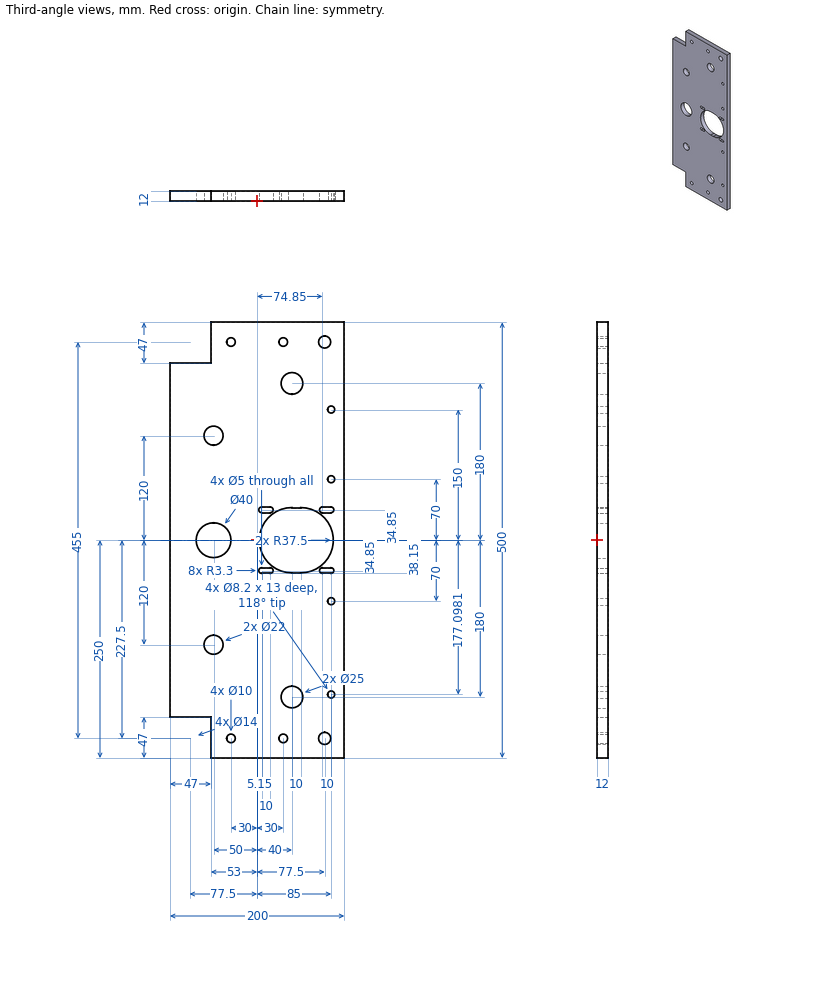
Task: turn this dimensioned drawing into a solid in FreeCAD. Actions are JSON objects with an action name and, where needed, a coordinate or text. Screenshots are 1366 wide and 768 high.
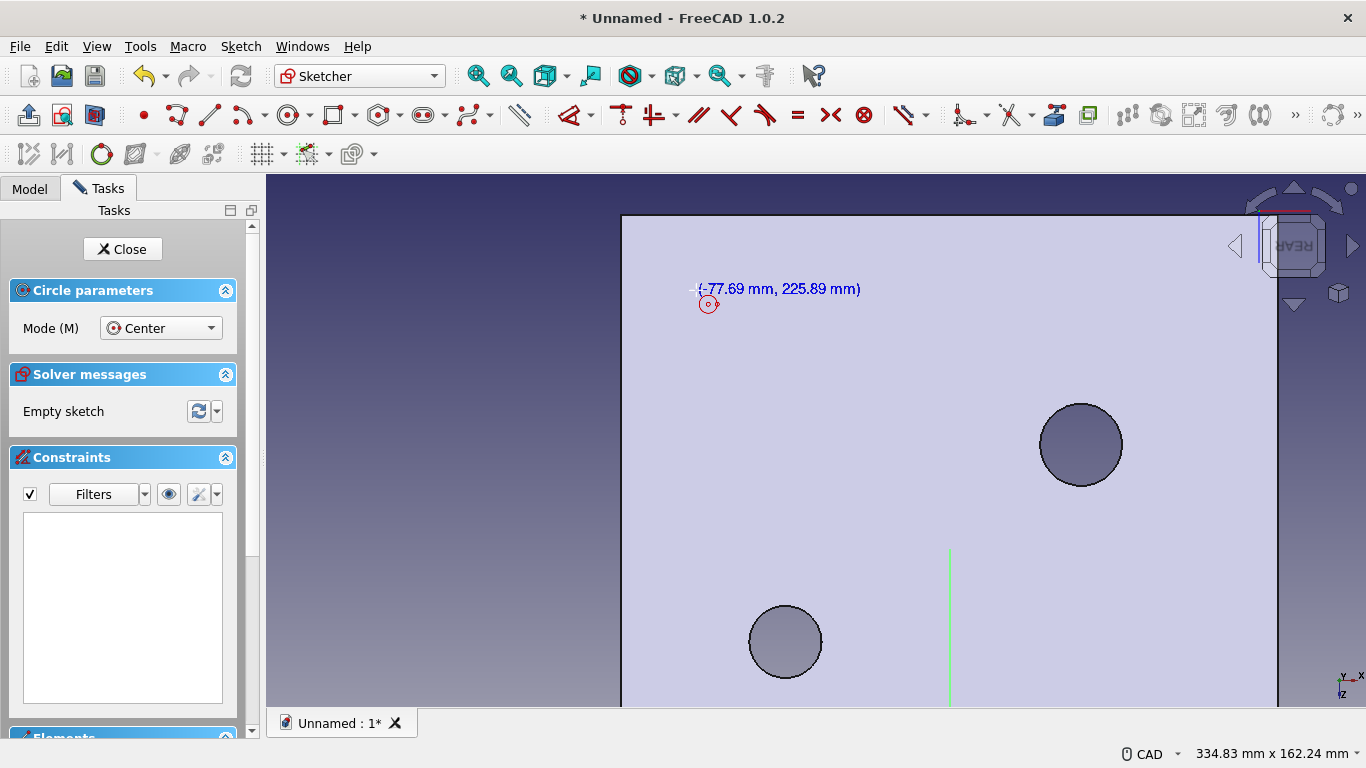
{"action": "scroll", "coordinate": [696, 290], "scroll_direction": "down", "scroll_amount": 8}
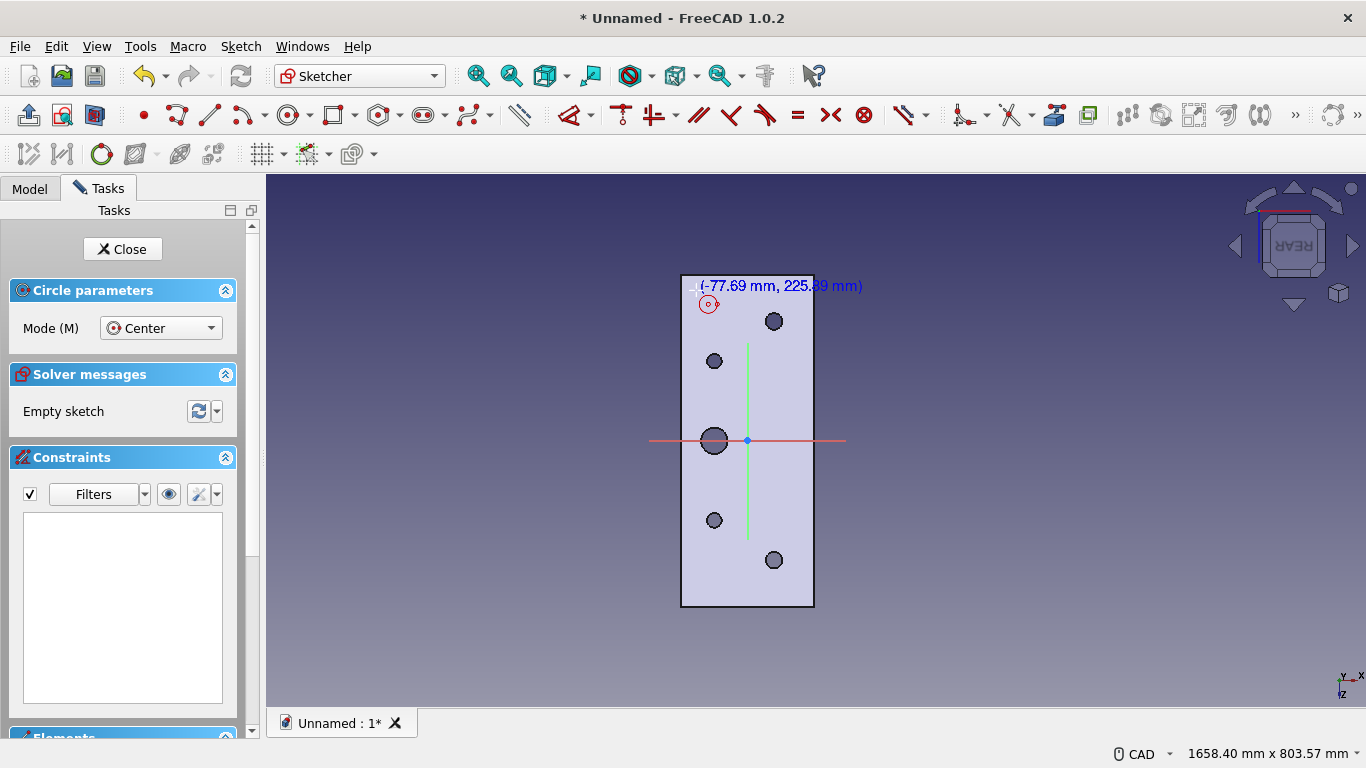
{"action": "left_click", "coordinate": [696, 290]}
{"action": "mouse_move", "coordinate": [699, 287]}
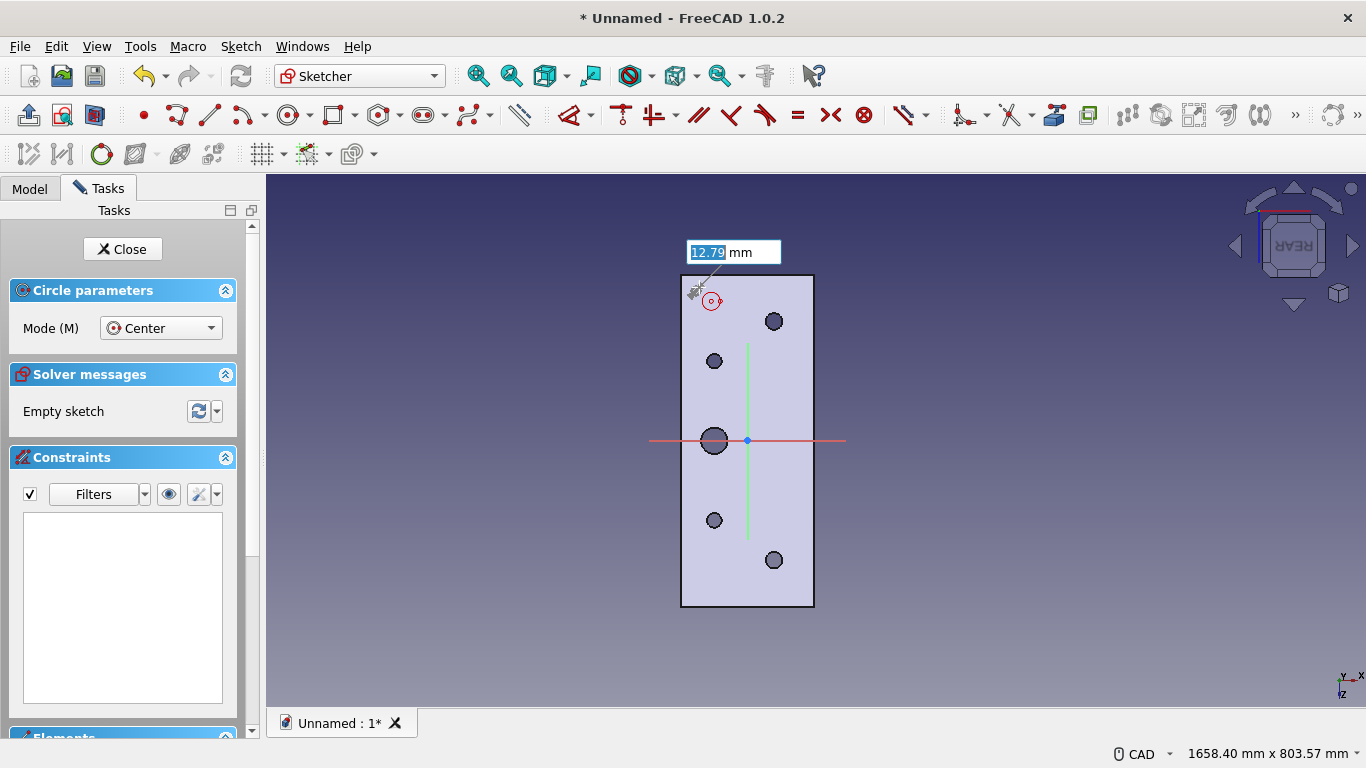
{"action": "type", "text": "14"}
{"action": "key", "text": "Return"}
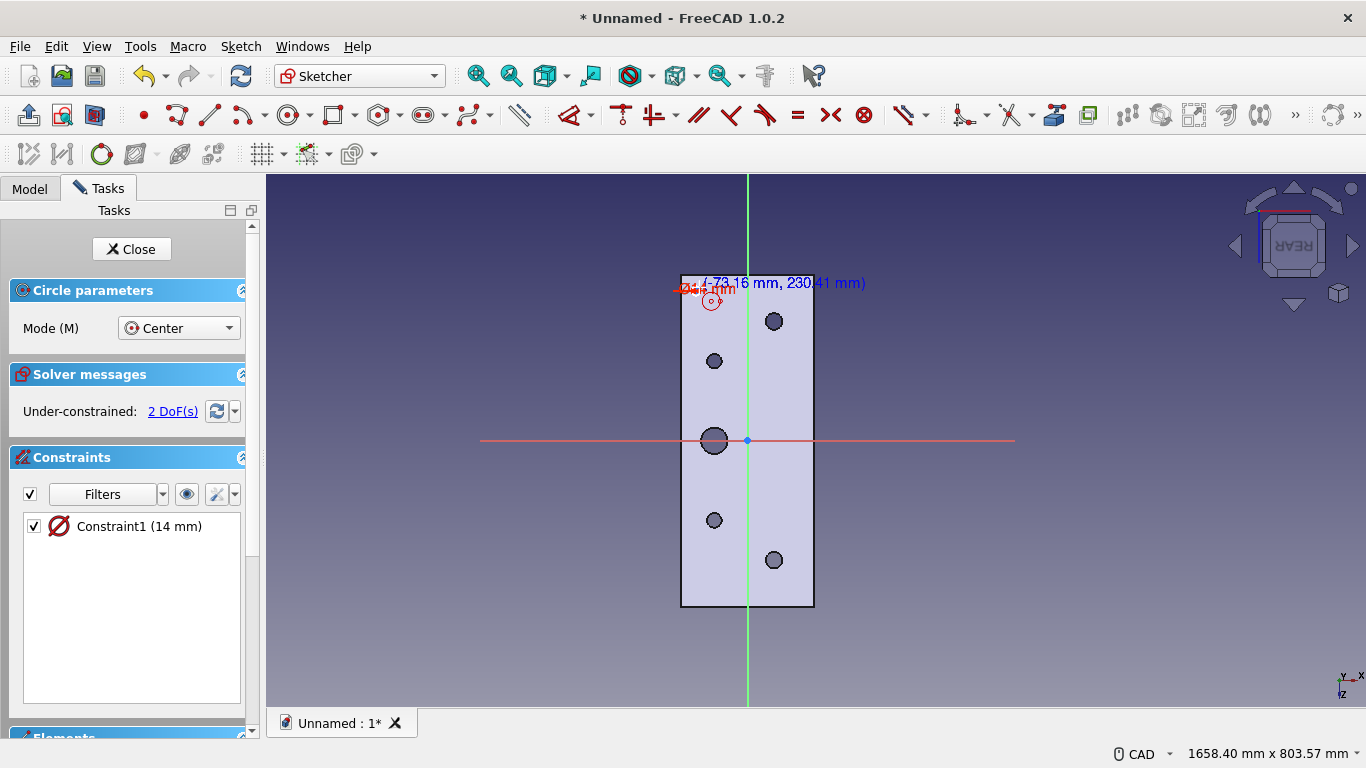
{"action": "scroll", "coordinate": [799, 290], "scroll_direction": "up", "scroll_amount": 8}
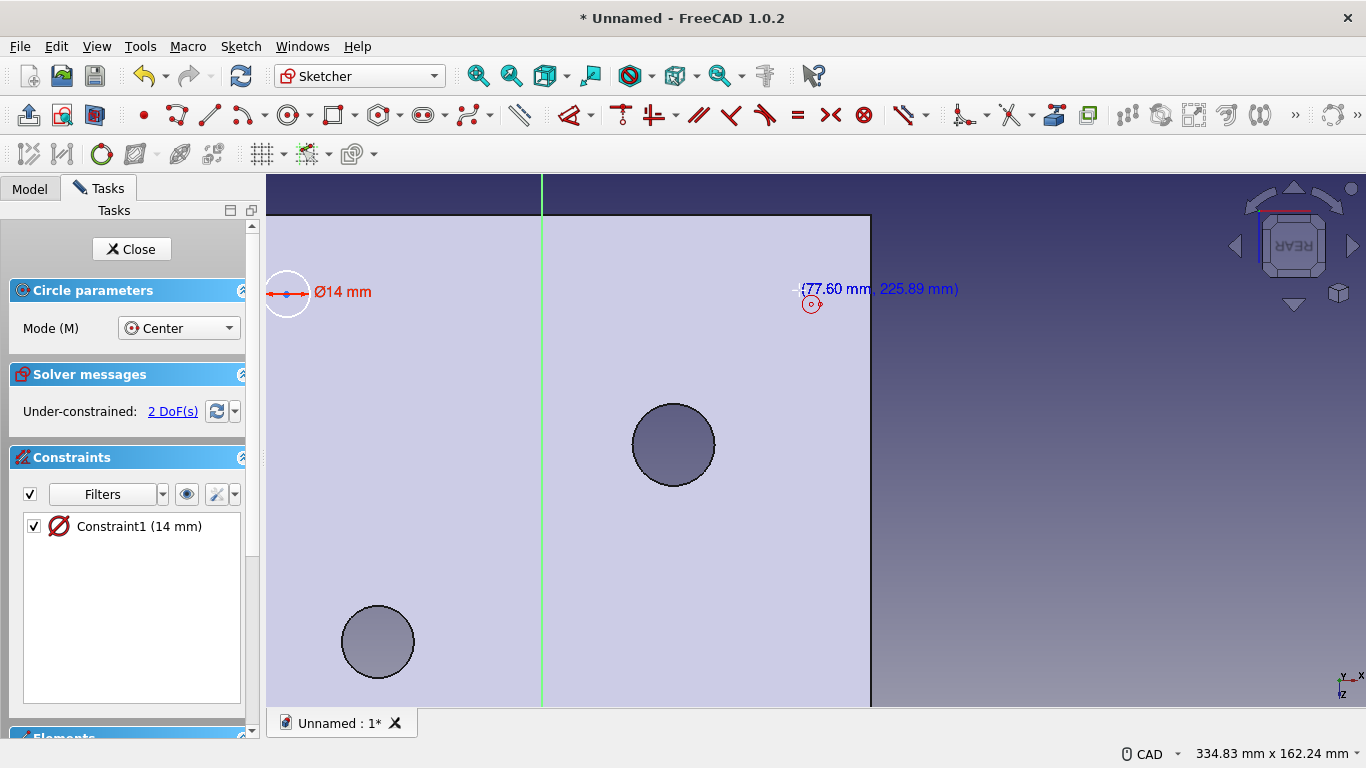
{"action": "scroll", "coordinate": [799, 290], "scroll_direction": "down", "scroll_amount": 8}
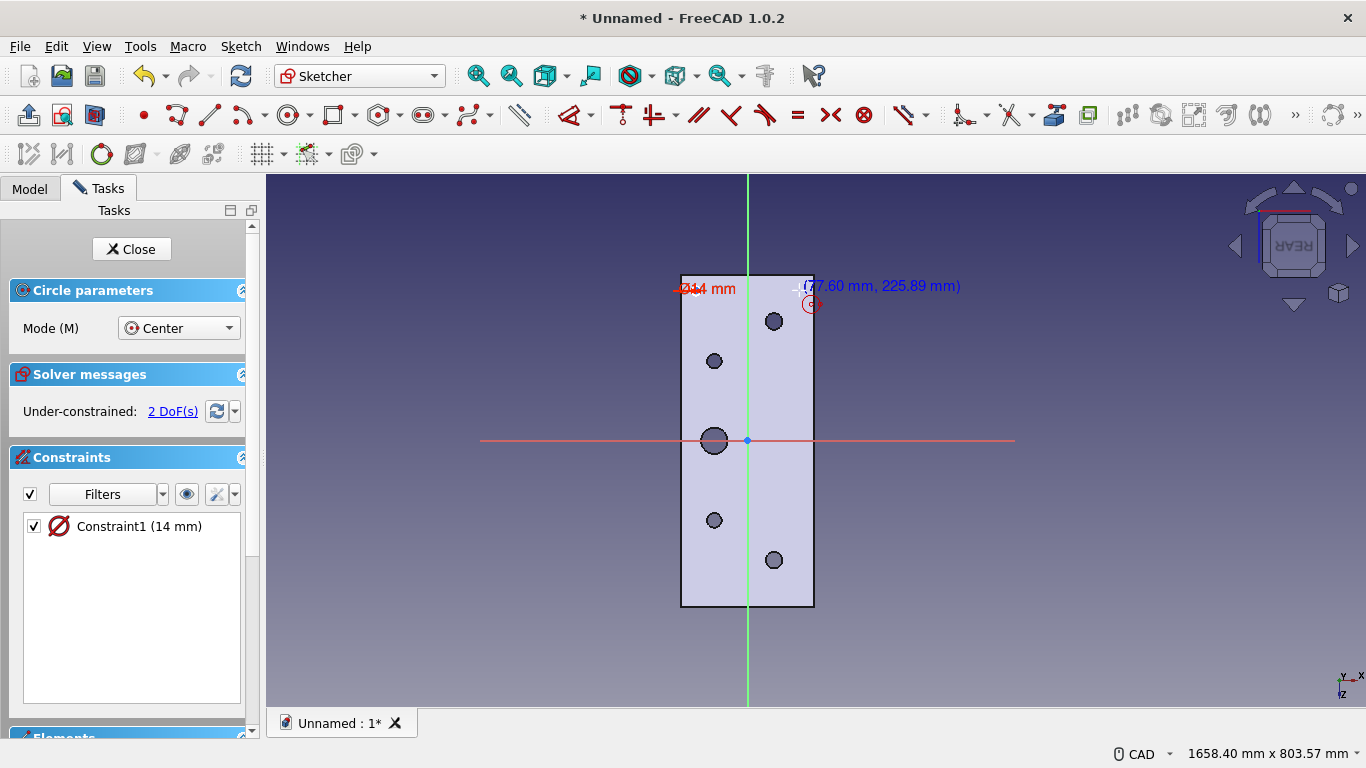
{"action": "left_click", "coordinate": [799, 290]}
{"action": "mouse_move", "coordinate": [802, 287]}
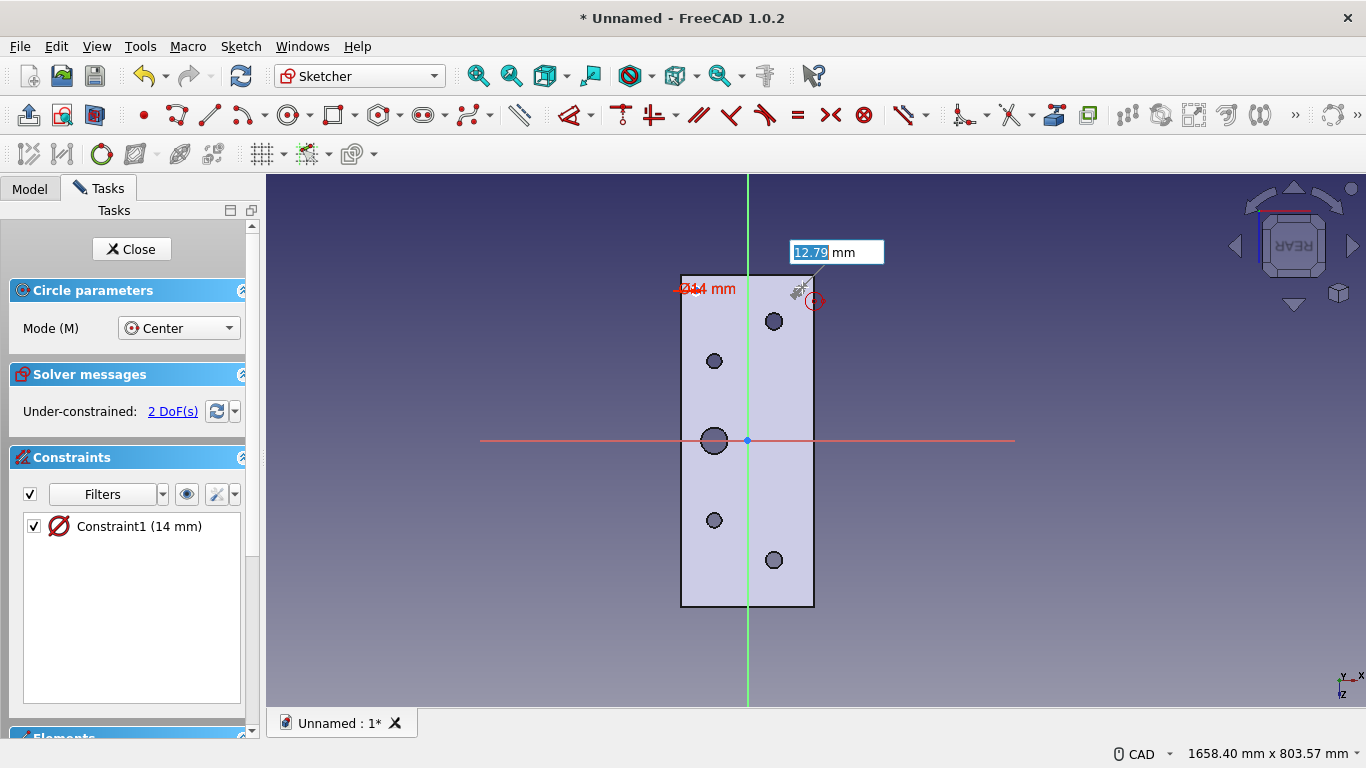
{"action": "type", "text": "14"}
{"action": "key", "text": "Return"}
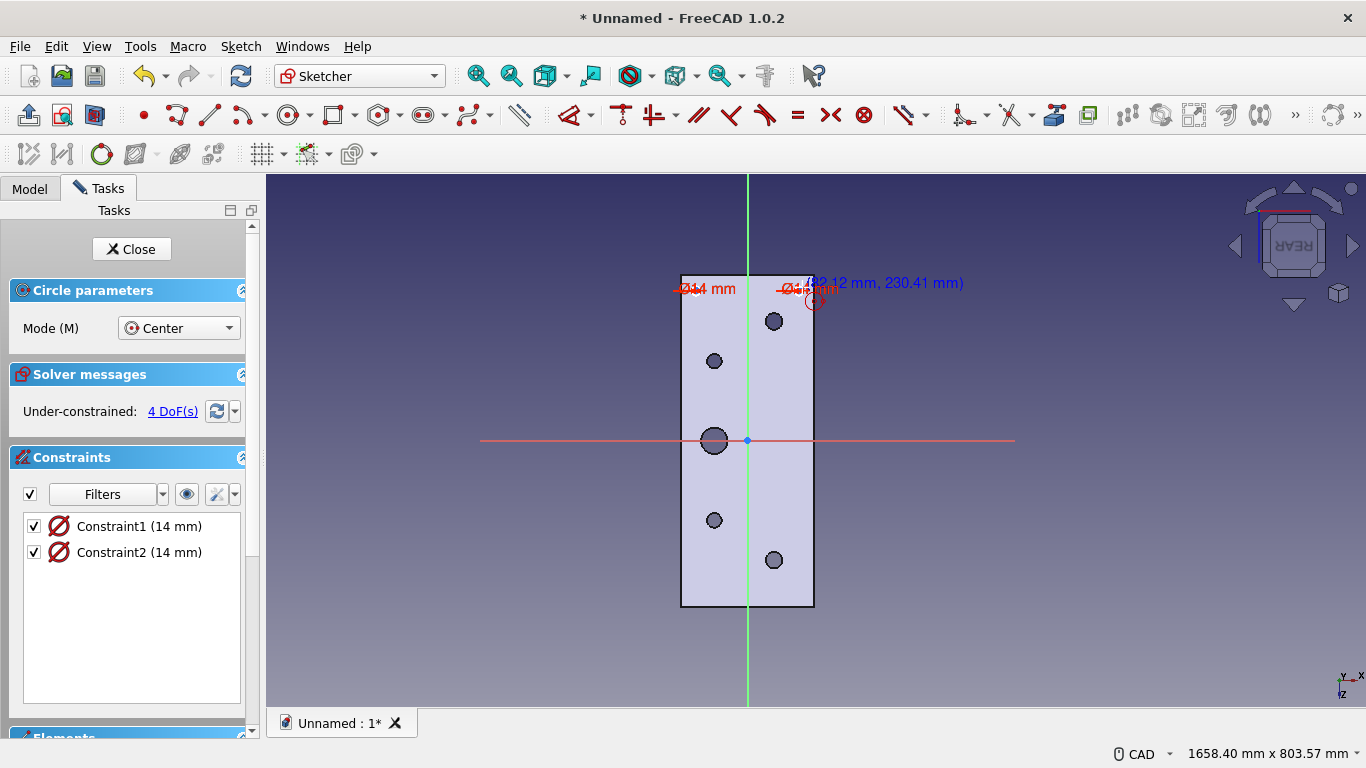
{"action": "scroll", "coordinate": [696, 592], "scroll_direction": "up", "scroll_amount": 8}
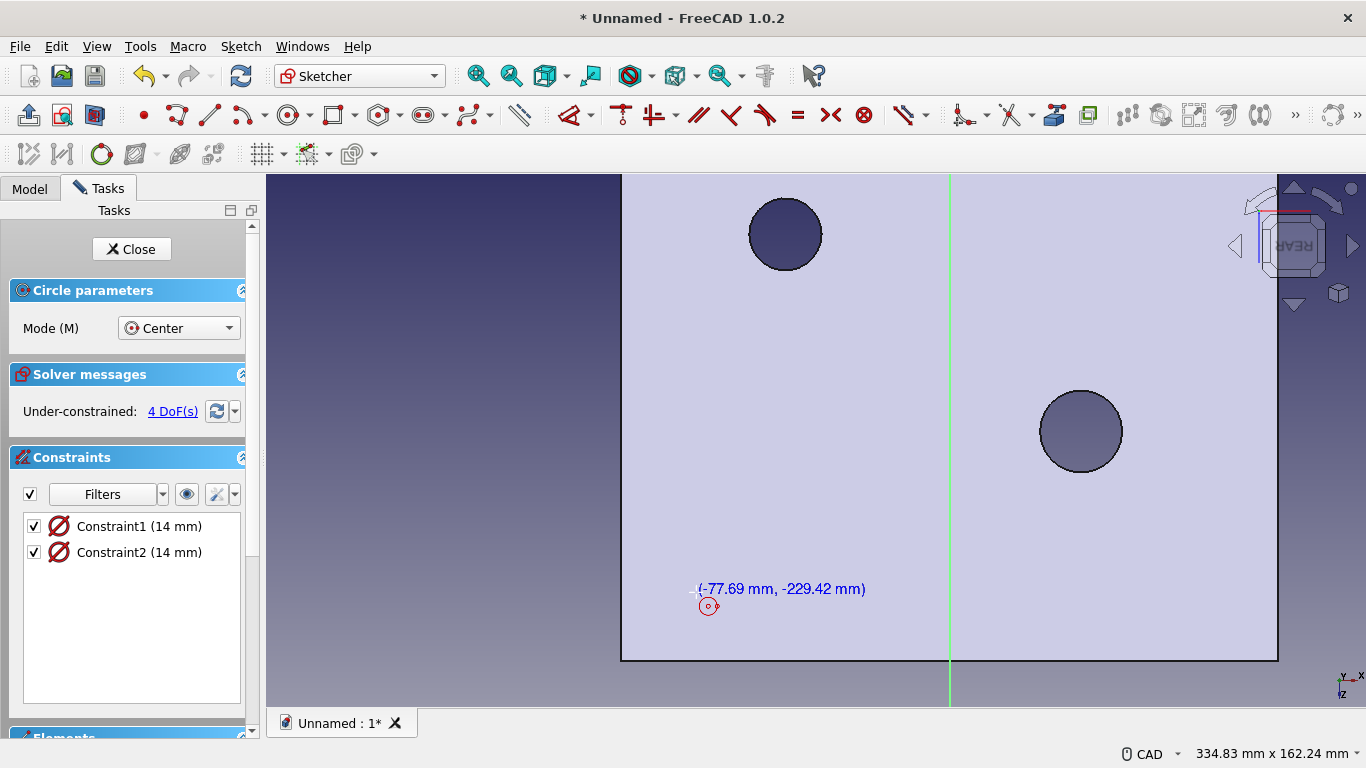
{"action": "scroll", "coordinate": [696, 592], "scroll_direction": "down", "scroll_amount": 8}